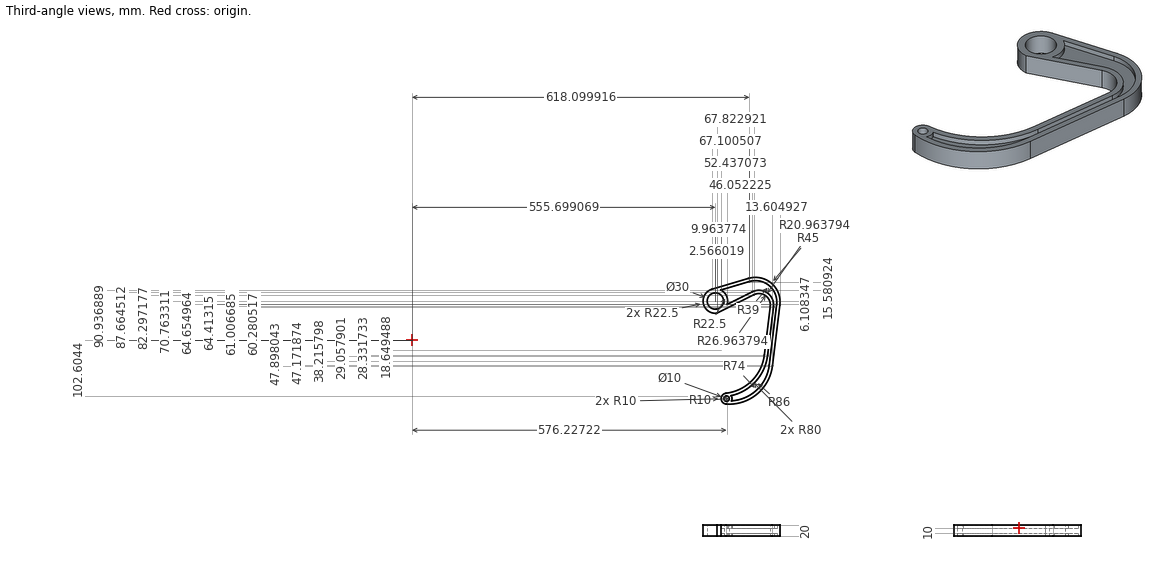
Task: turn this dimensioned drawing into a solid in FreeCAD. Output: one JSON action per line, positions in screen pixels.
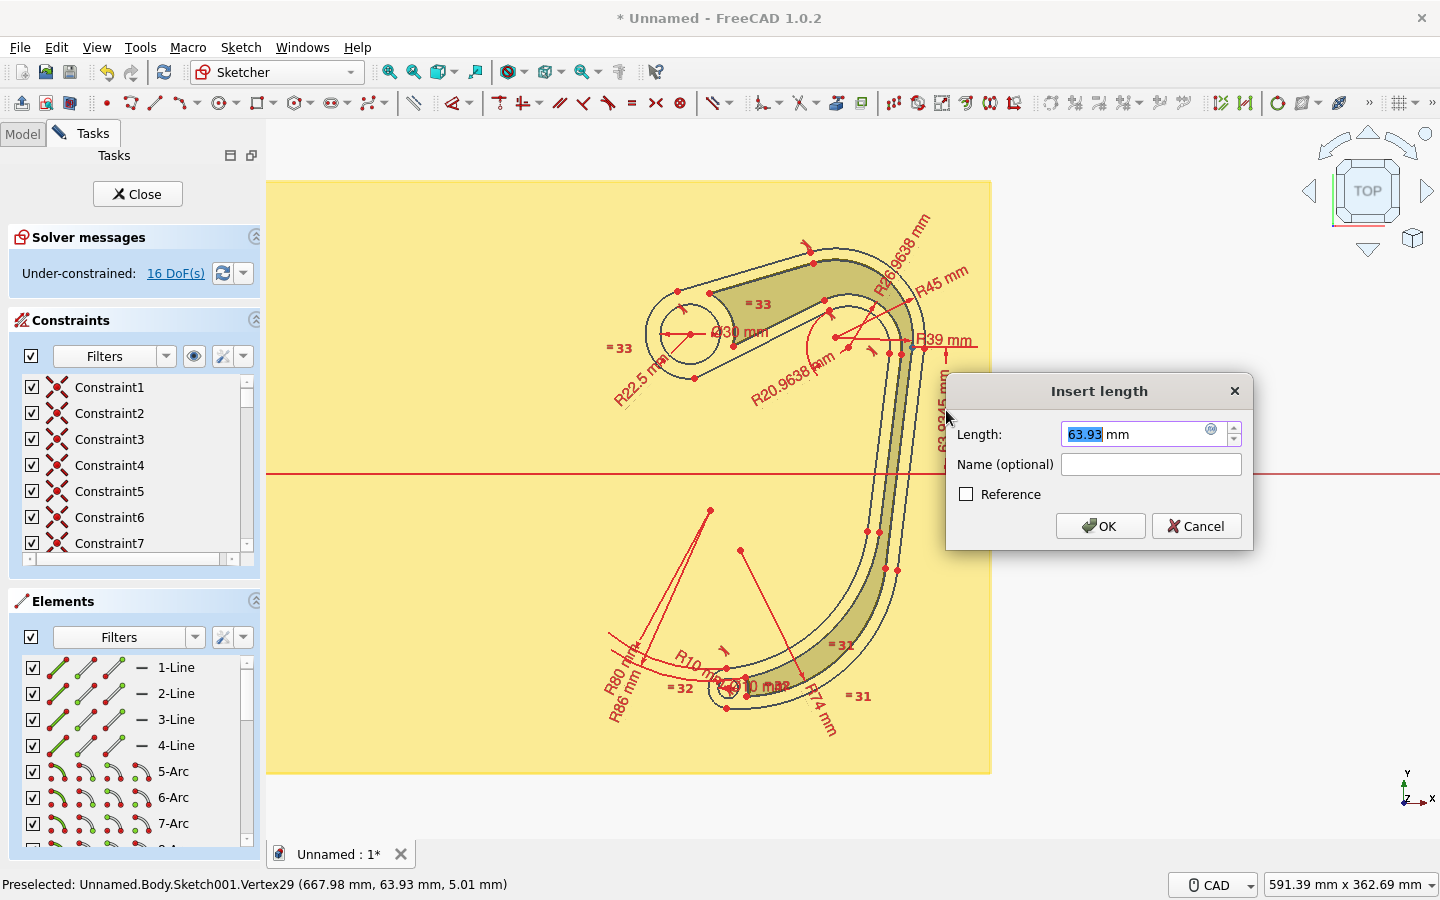
{"action": "type", "text": "64.41315"}
{"action": "key", "text": "Return"}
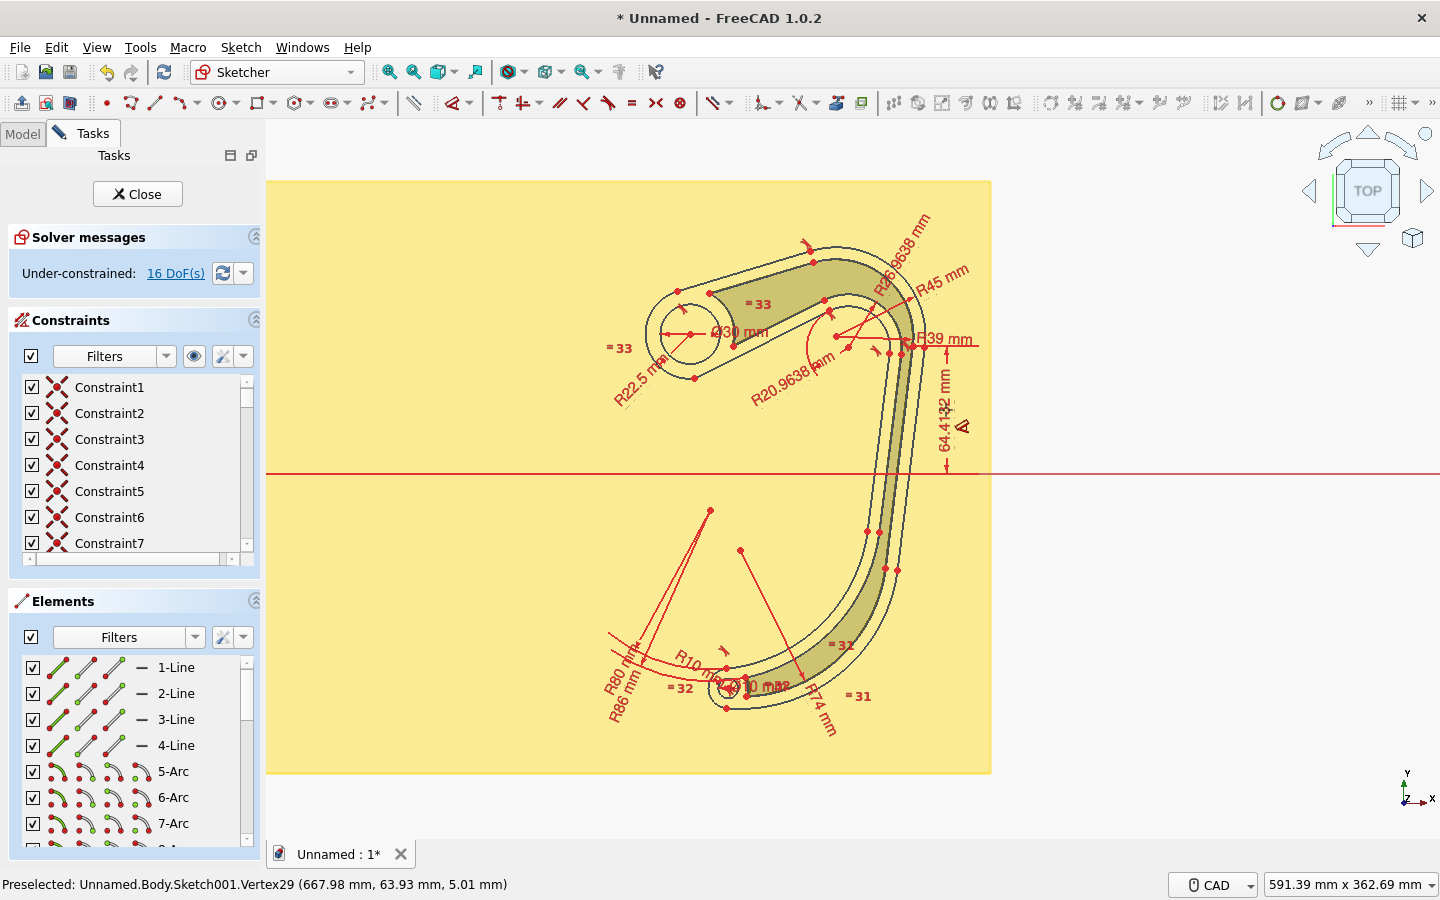
{"action": "left_click", "coordinate": [745, 678]}
{"action": "left_click", "coordinate": [779, 576]}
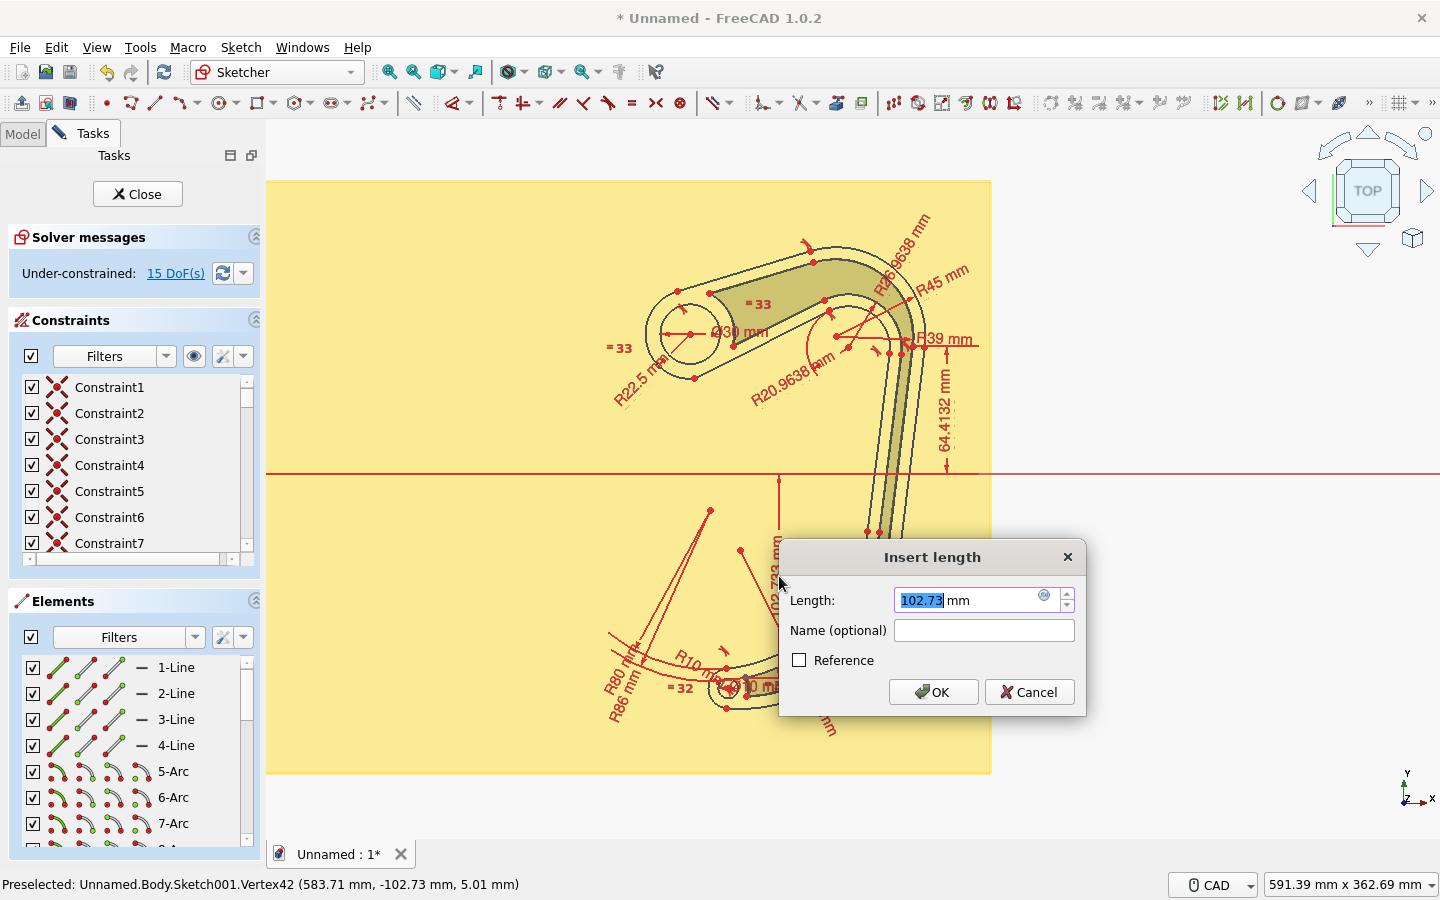
{"action": "type", "text": "102.6044"}
{"action": "key", "text": "Return"}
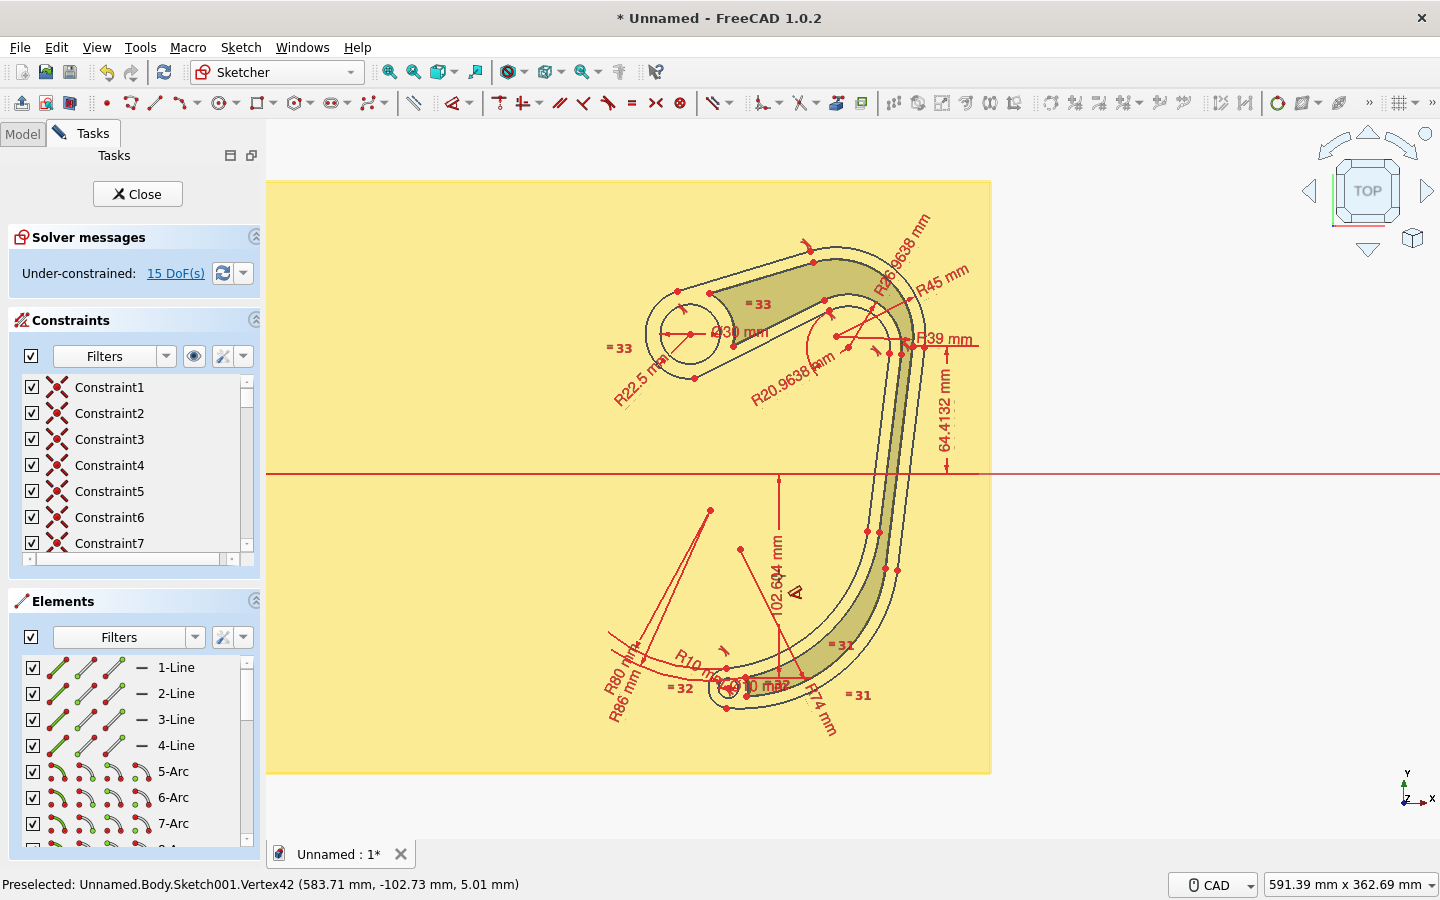
{"action": "left_click", "coordinate": [728, 688]}
{"action": "left_click", "coordinate": [511, 722]}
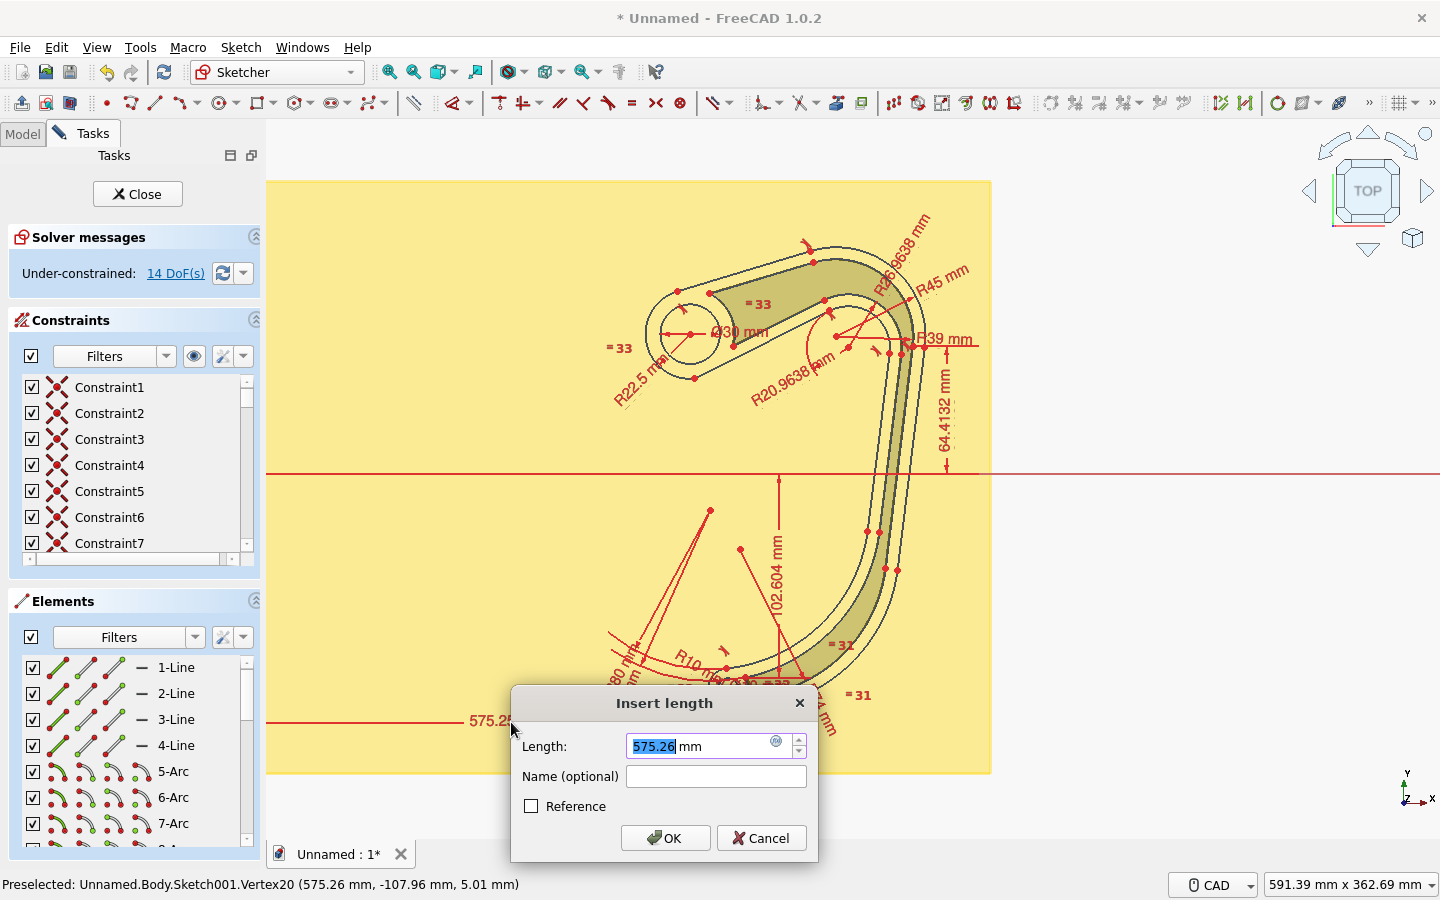
{"action": "type", "text": "576.22722"}
{"action": "key", "text": "Return"}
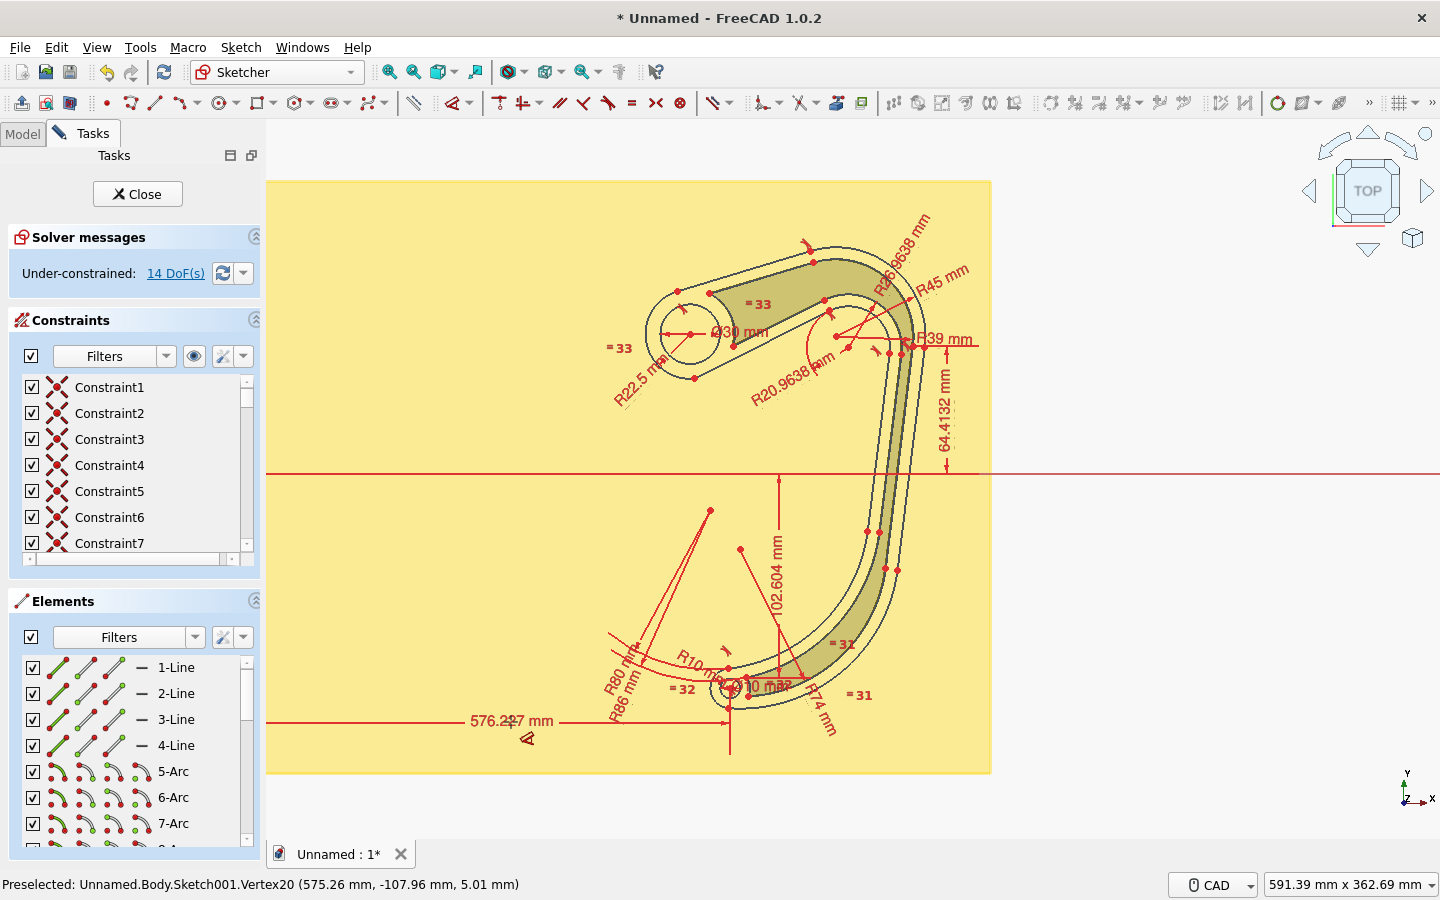
{"action": "left_click", "coordinate": [690, 334]}
{"action": "left_click", "coordinate": [724, 404]}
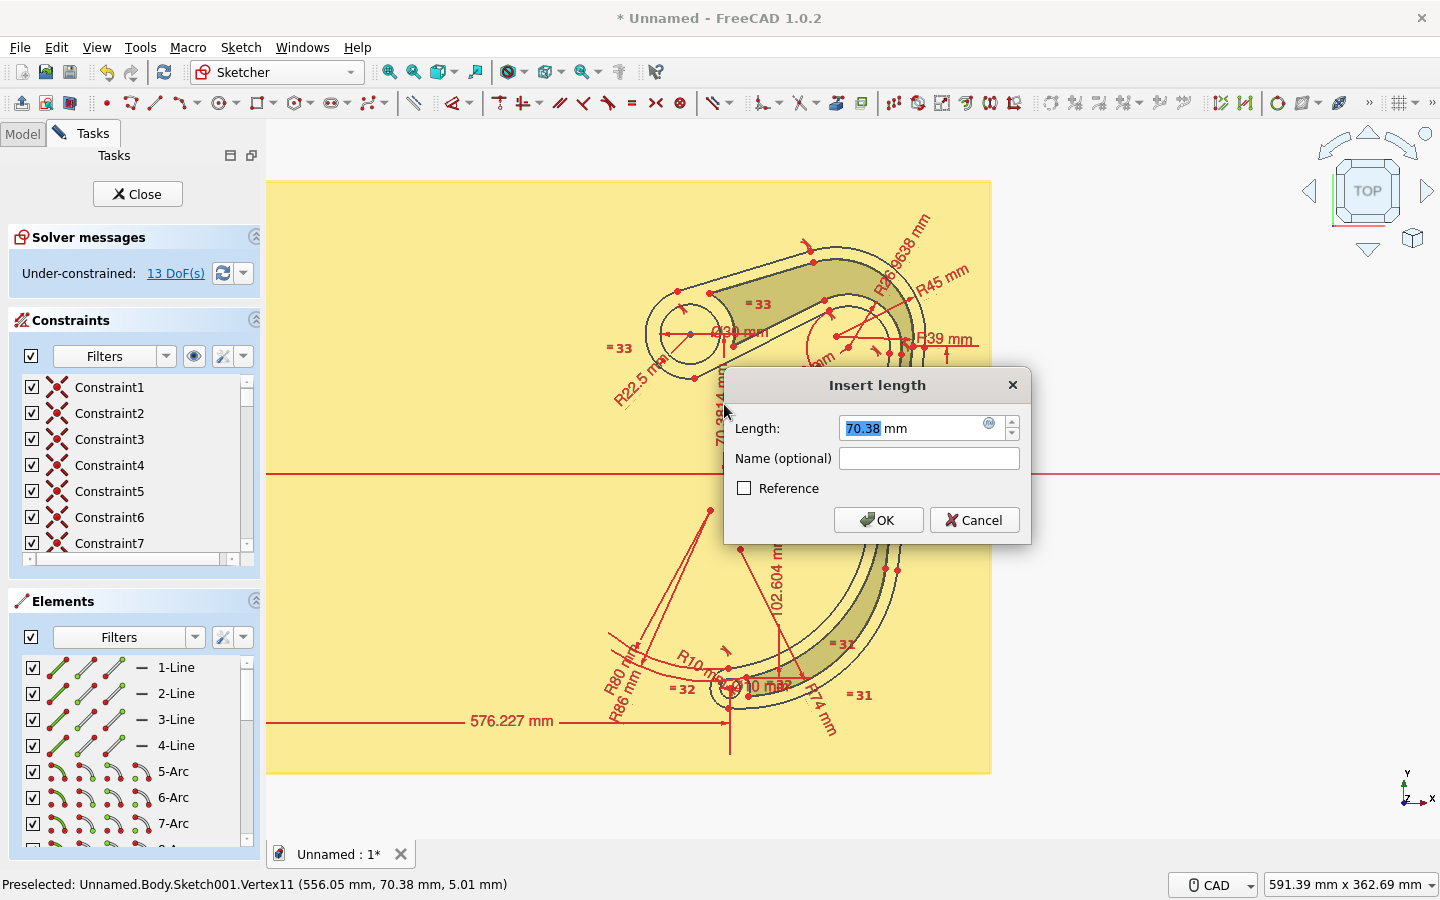
{"action": "type", "text": "70.763311"}
{"action": "key", "text": "Return"}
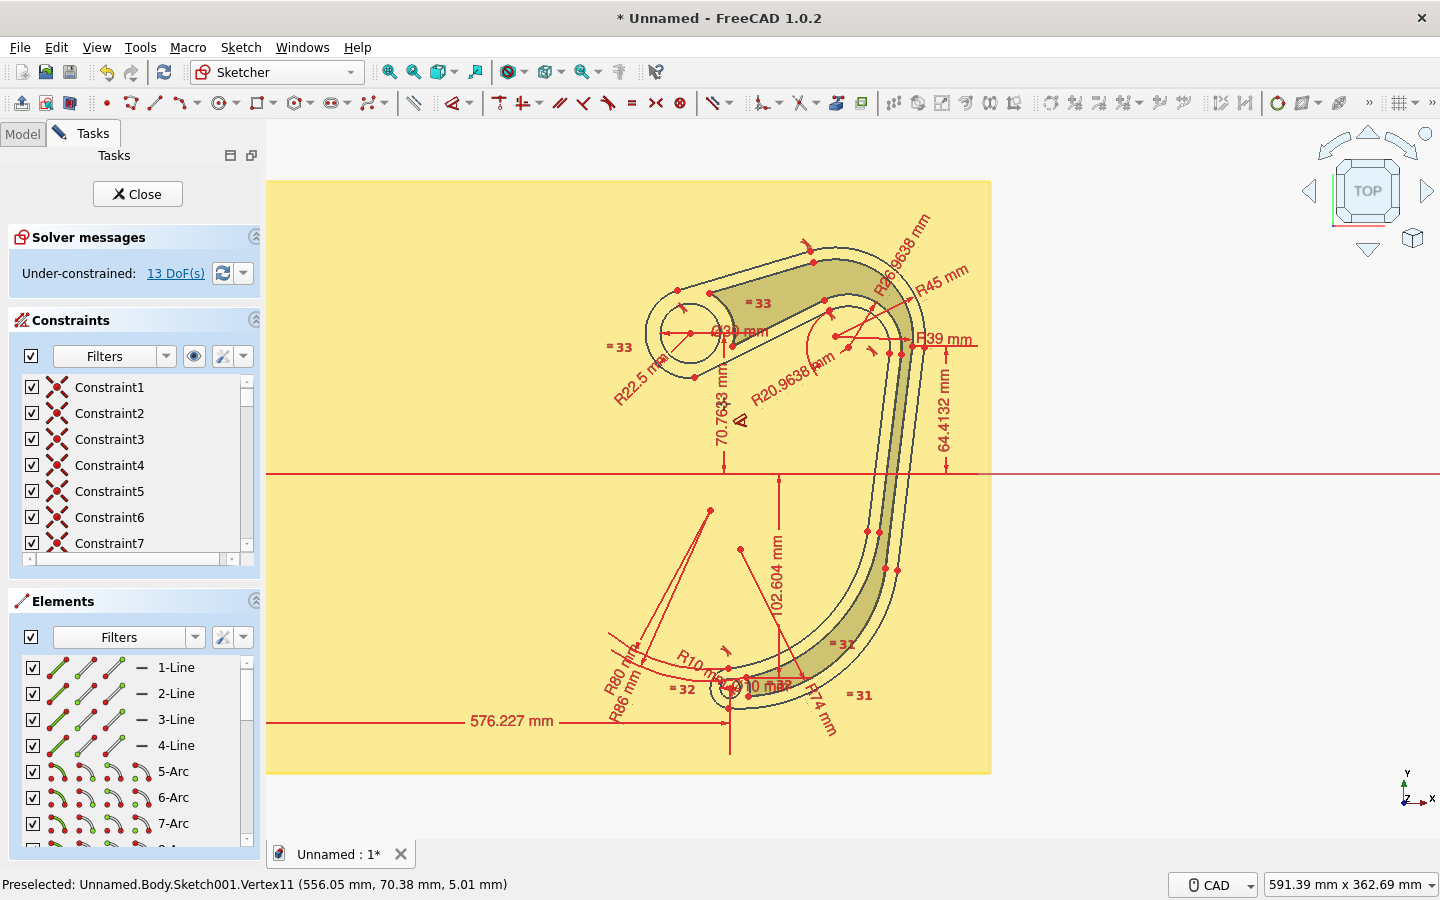
{"action": "scroll", "coordinate": [710, 293], "scroll_direction": "up", "scroll_amount": 4}